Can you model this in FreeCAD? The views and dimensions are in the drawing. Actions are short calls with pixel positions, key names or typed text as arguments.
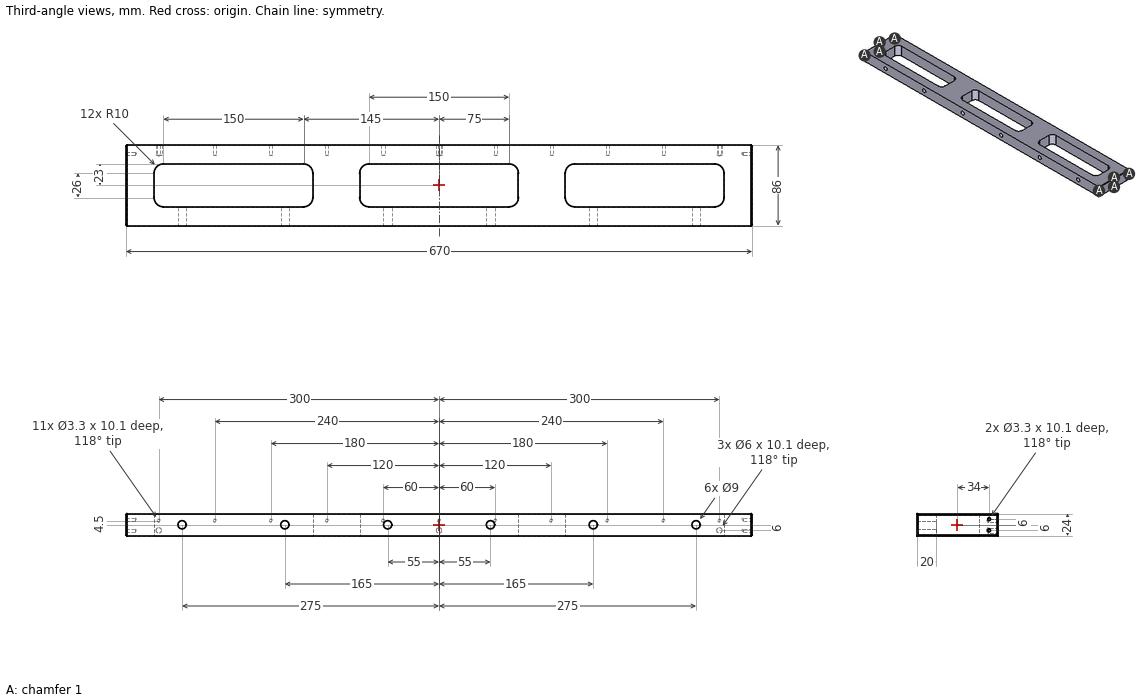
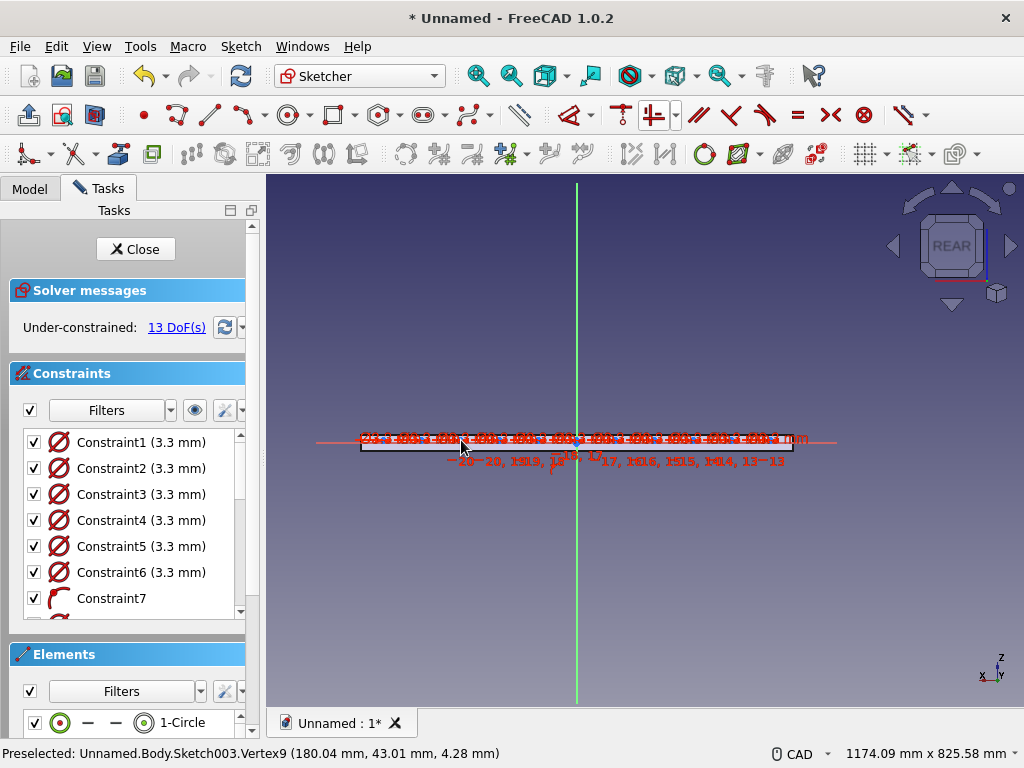
click(461, 440)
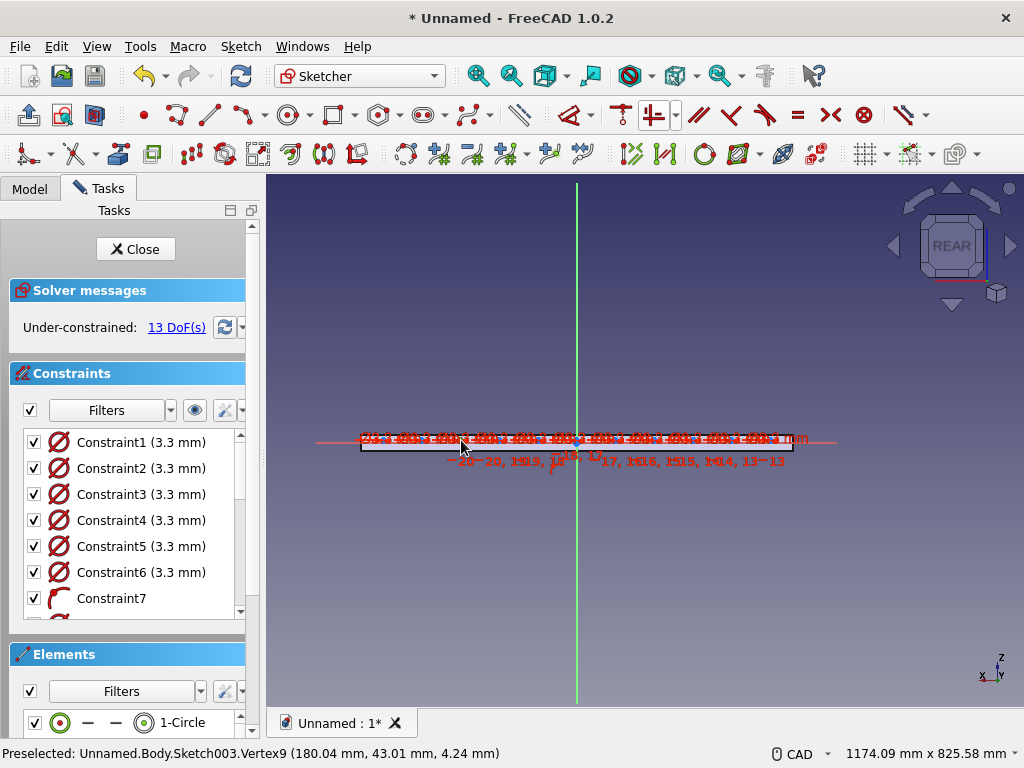
click(422, 440)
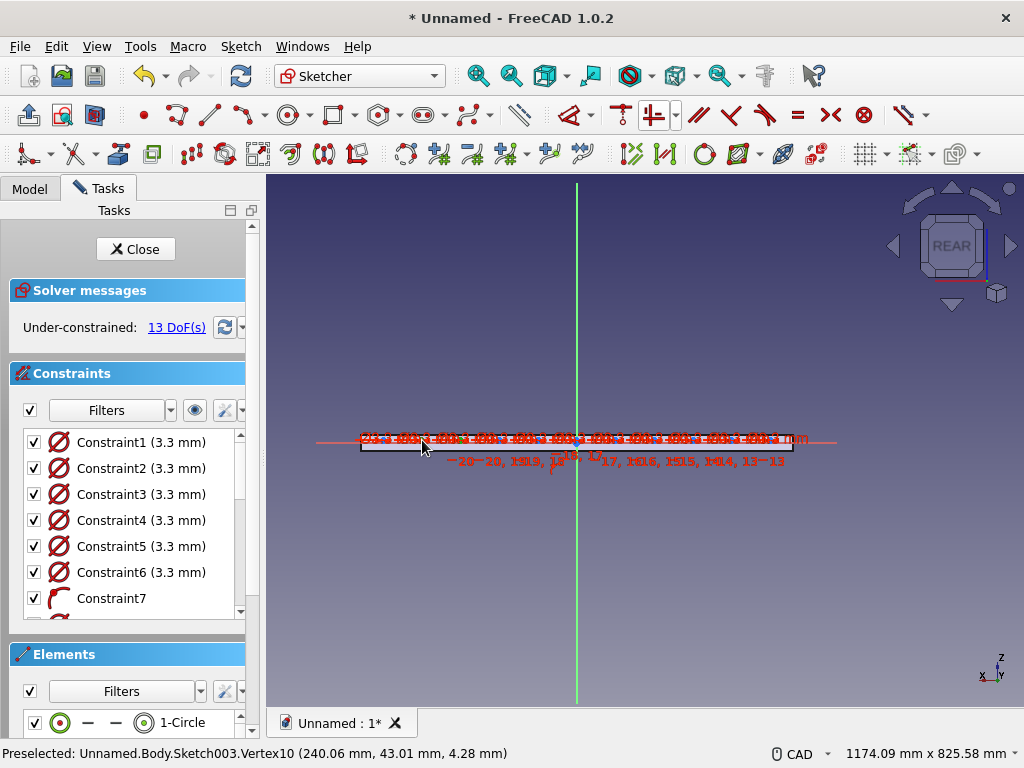
key(h)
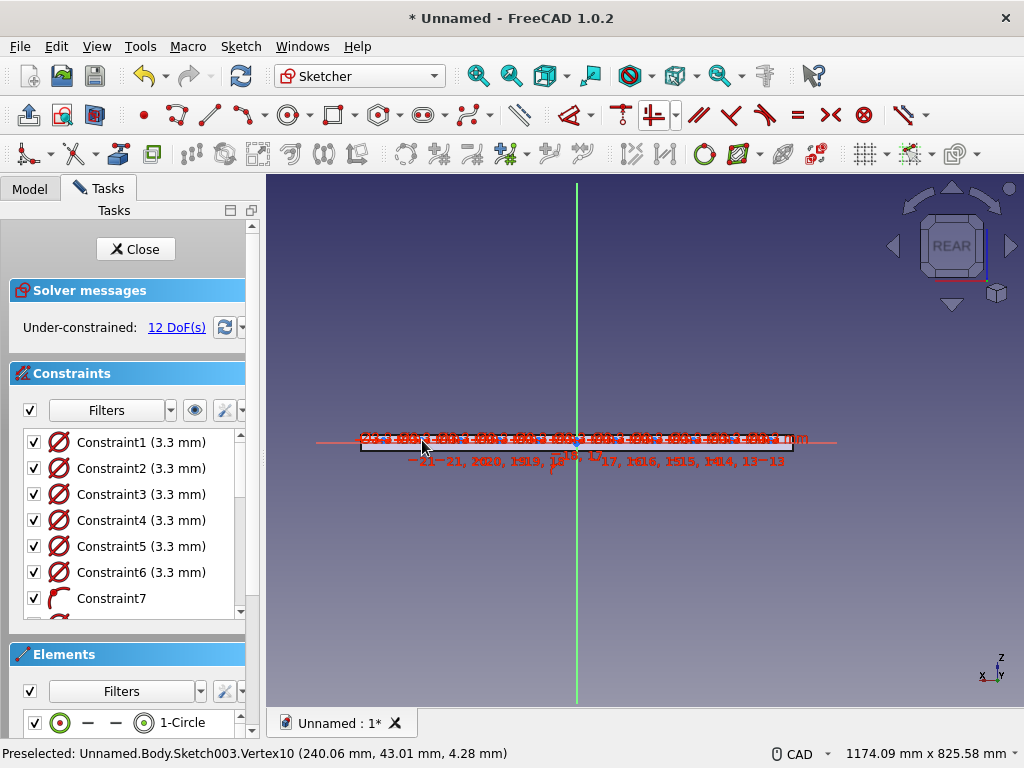
click(422, 440)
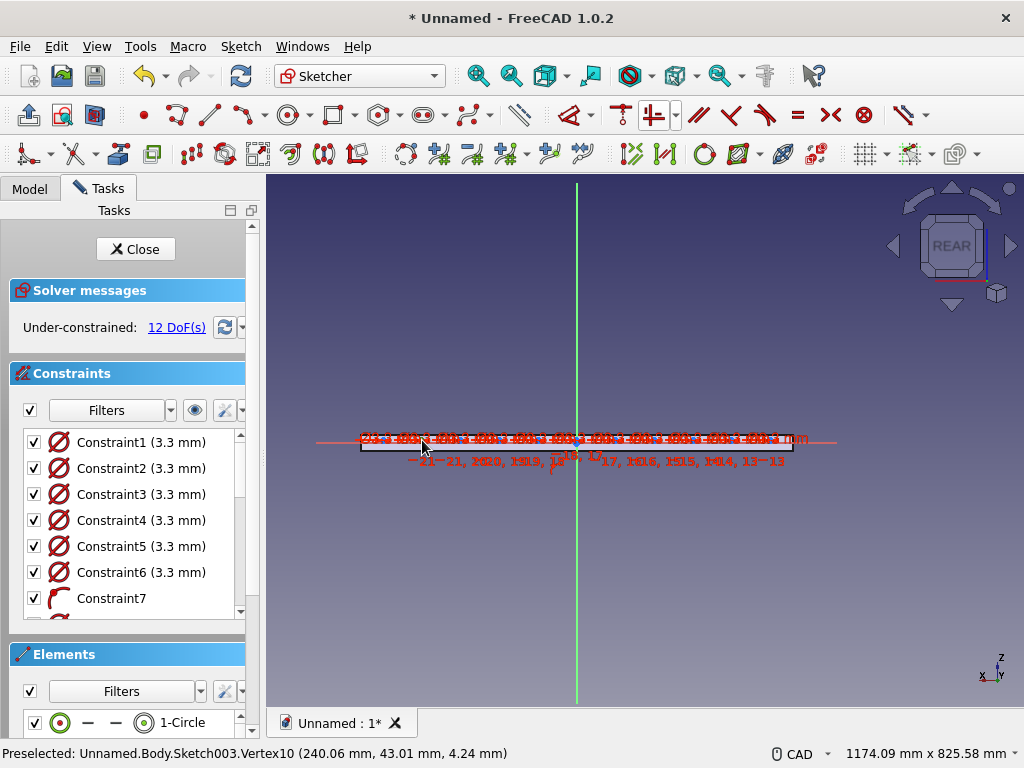
click(383, 440)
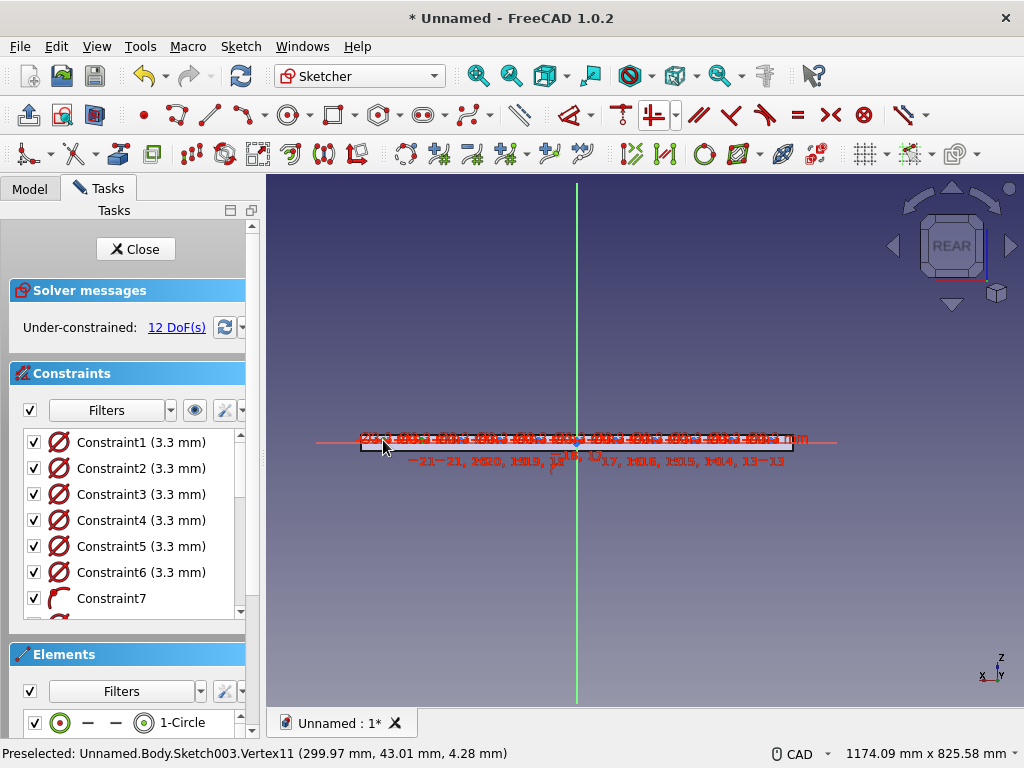
key(h)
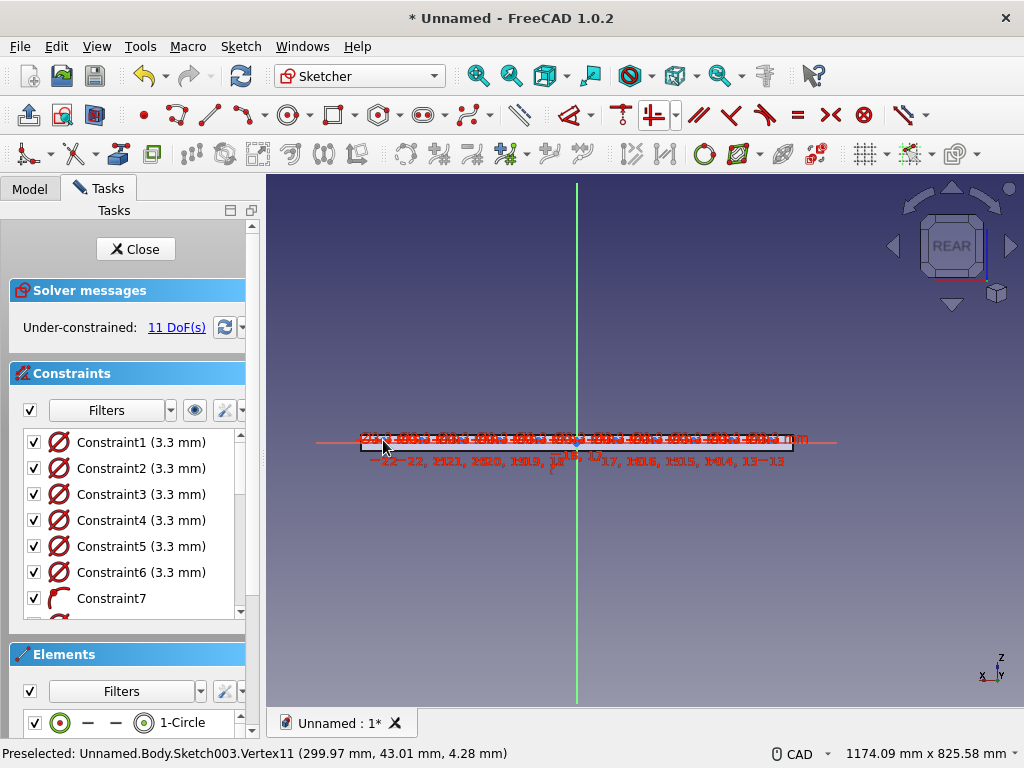
click(568, 116)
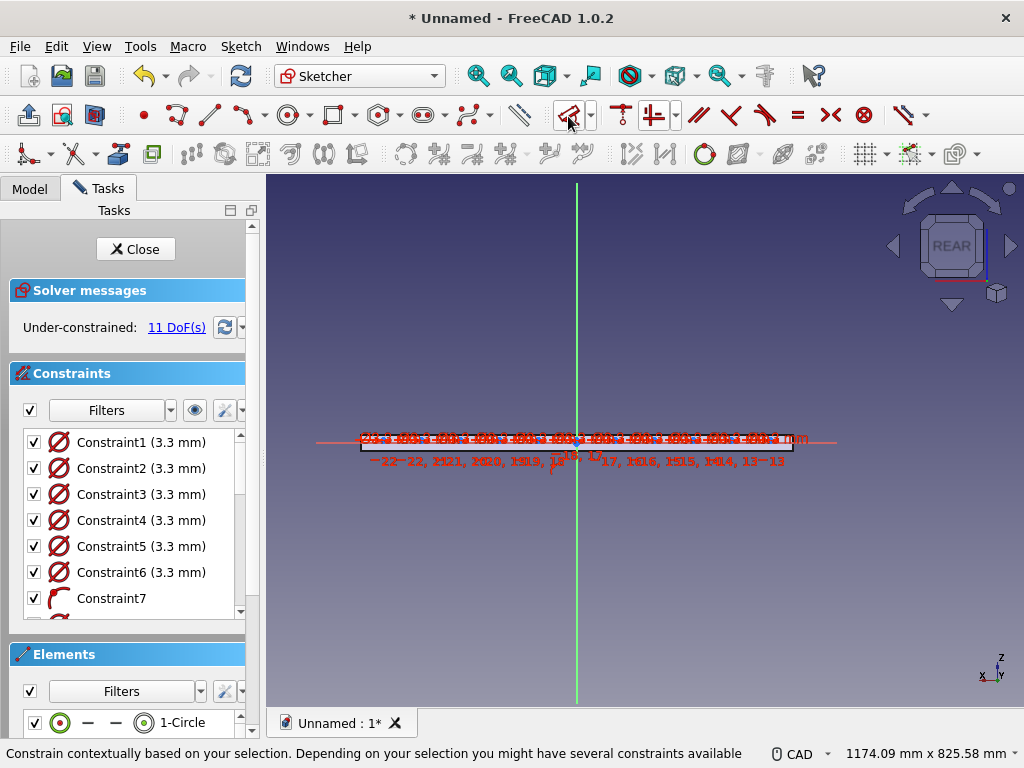
click(616, 440)
click(596, 477)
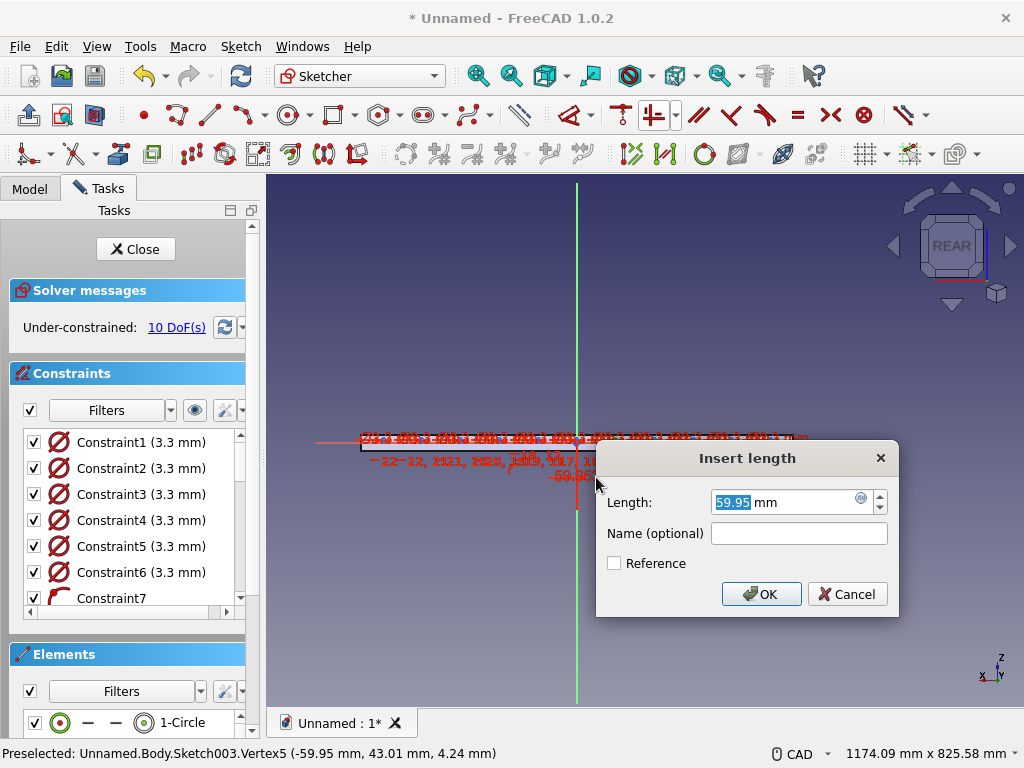
text(60)
key(Return)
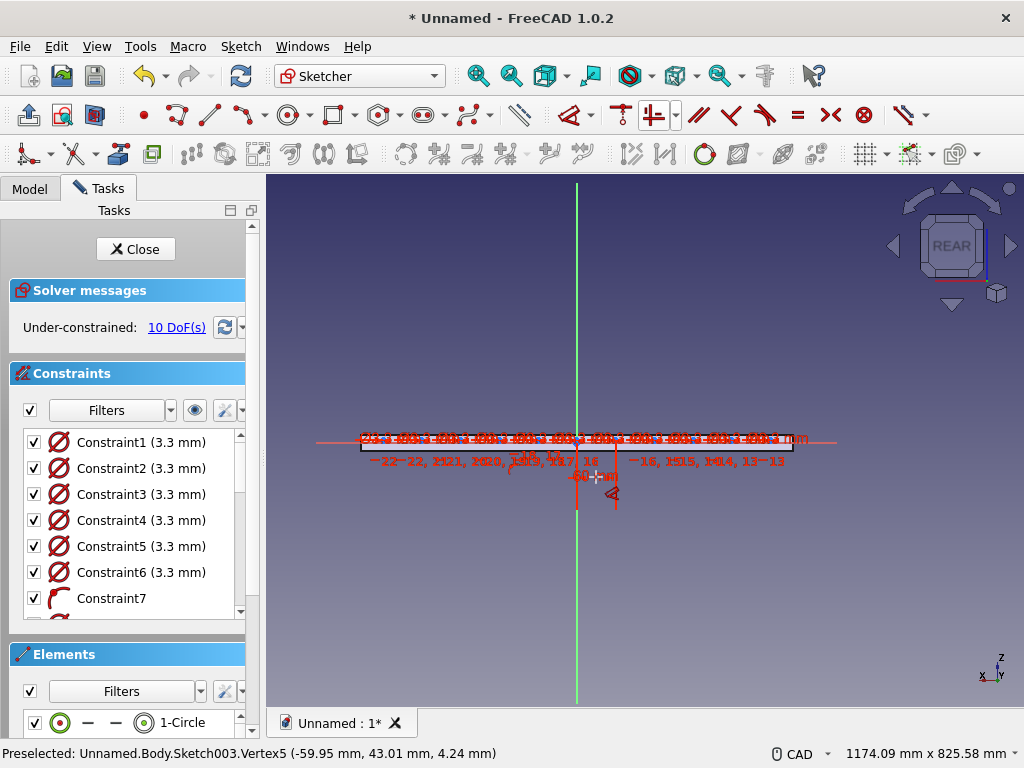
click(538, 440)
click(558, 406)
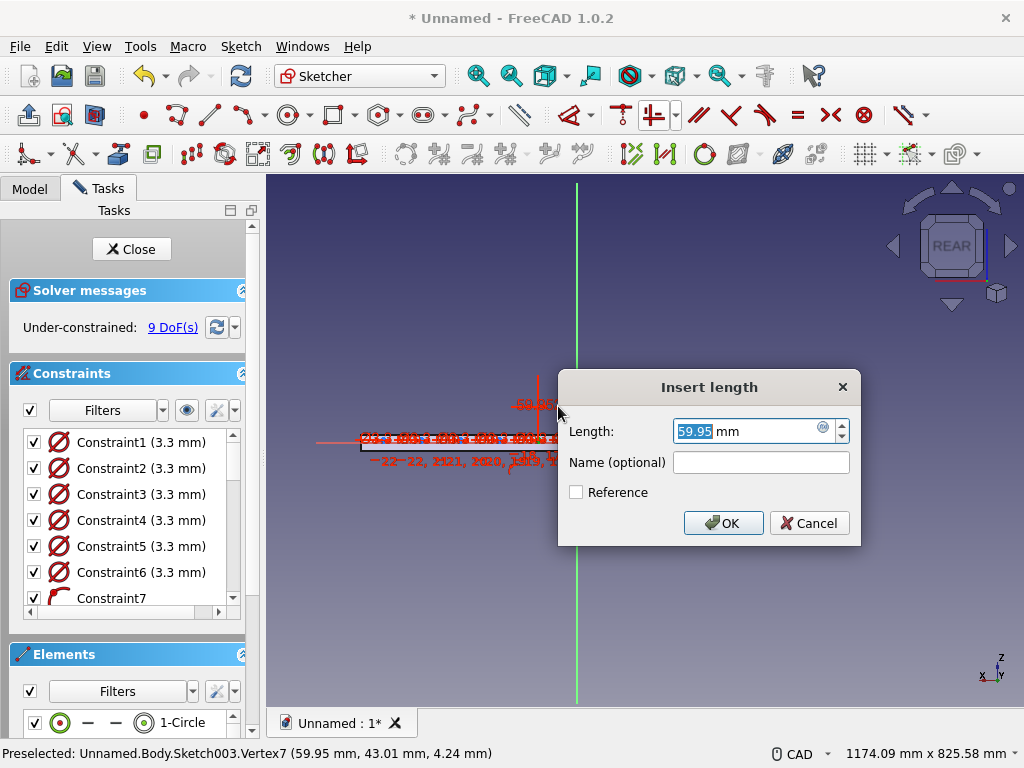
text(60)
key(Return)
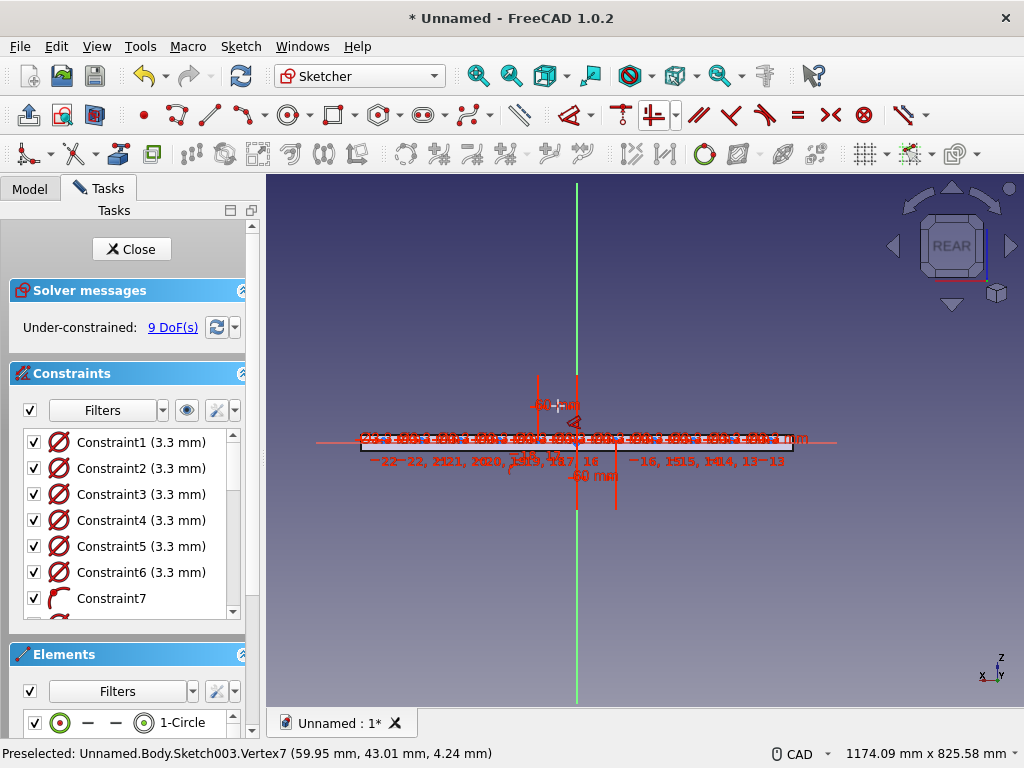
click(771, 440)
click(674, 477)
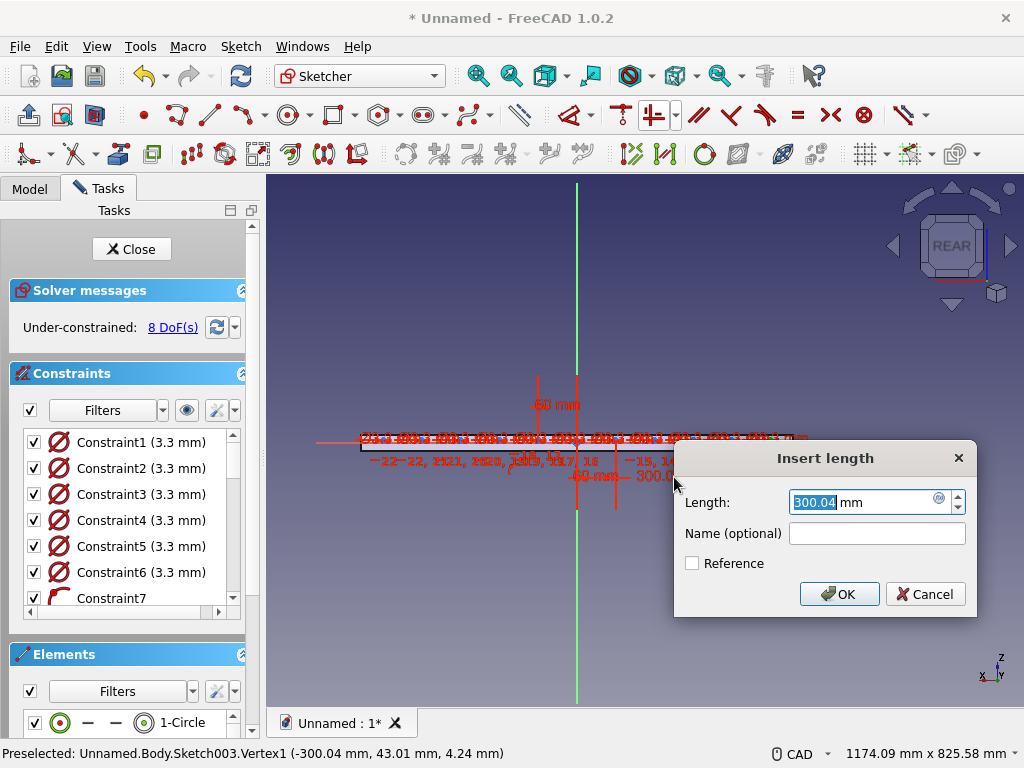
text(300)
key(Return)